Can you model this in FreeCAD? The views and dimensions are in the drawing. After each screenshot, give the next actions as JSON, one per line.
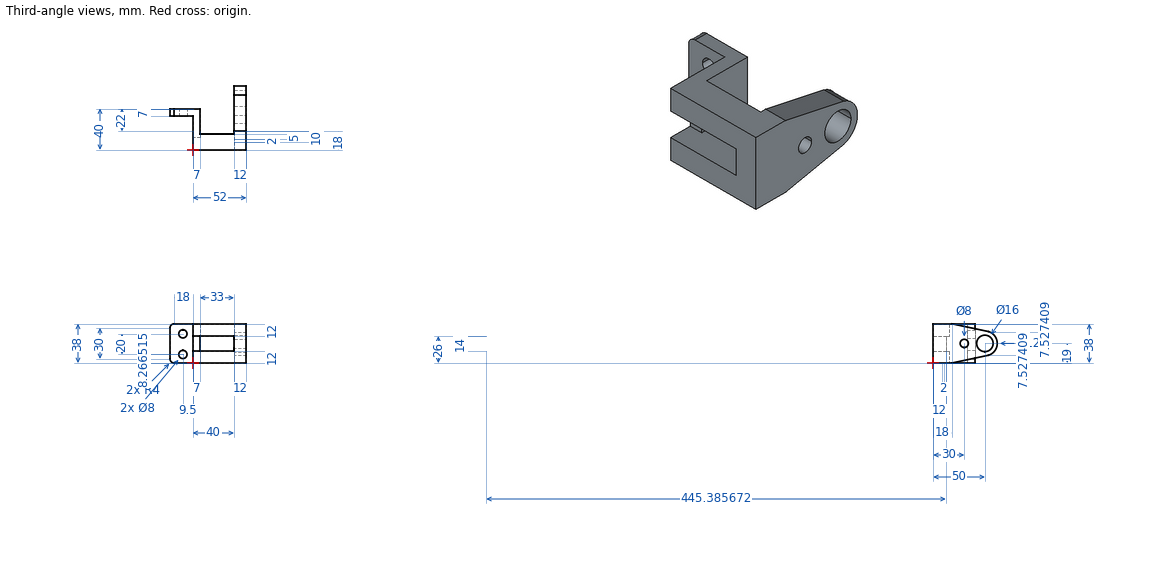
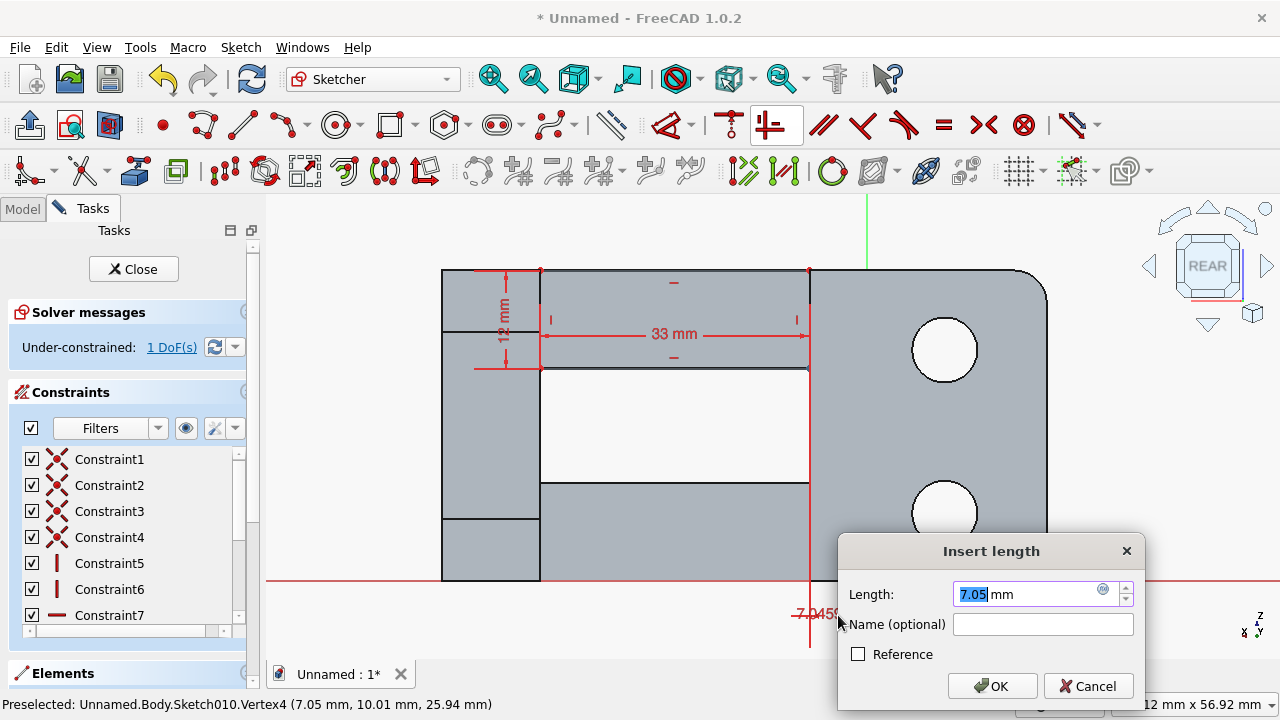
{"action": "type", "text": "7"}
{"action": "key", "text": "Return"}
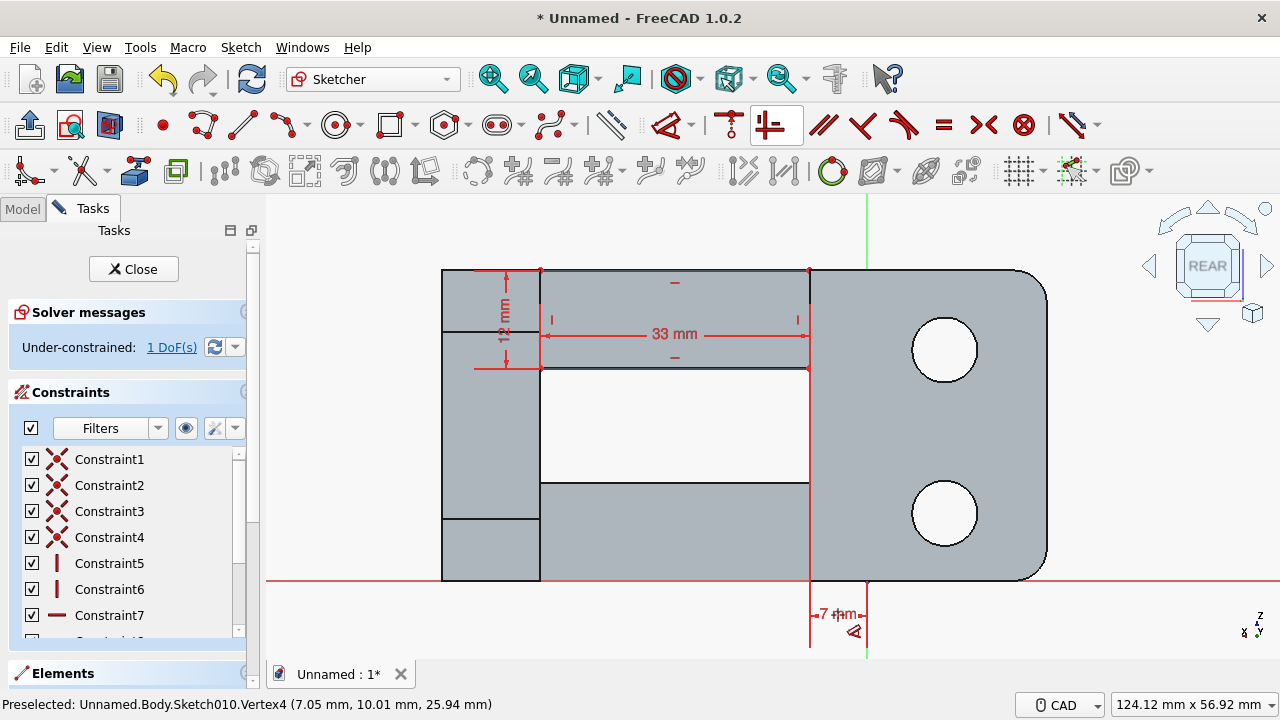
{"action": "left_click", "coordinate": [540, 271]}
{"action": "left_click", "coordinate": [506, 426]}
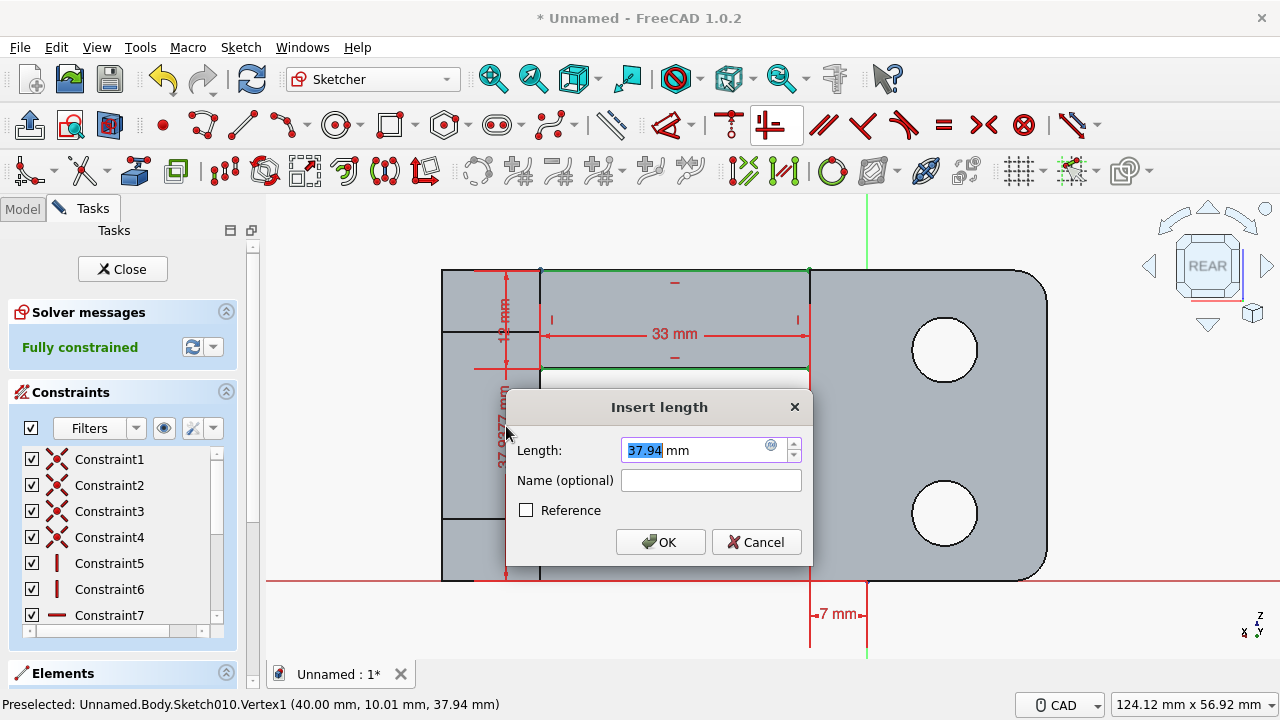
{"action": "type", "text": "38"}
{"action": "key", "text": "Return"}
{"action": "key", "text": "Escape"}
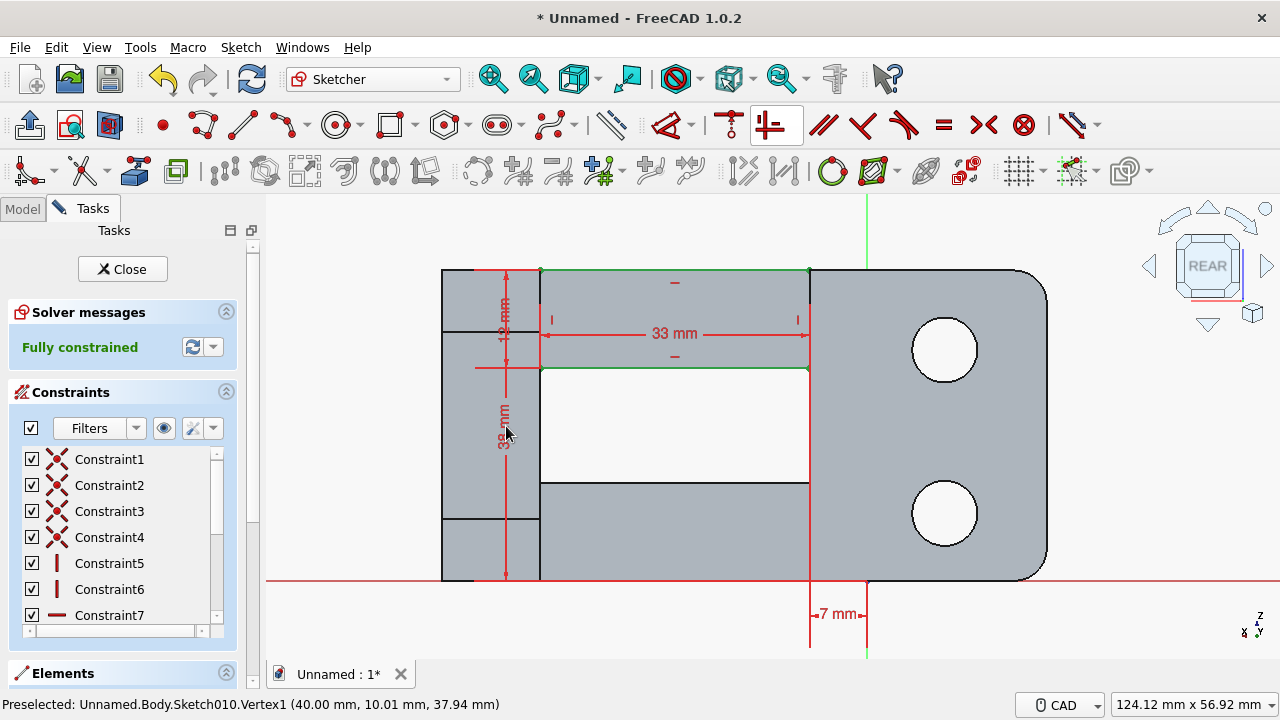
{"action": "left_click", "coordinate": [123, 269]}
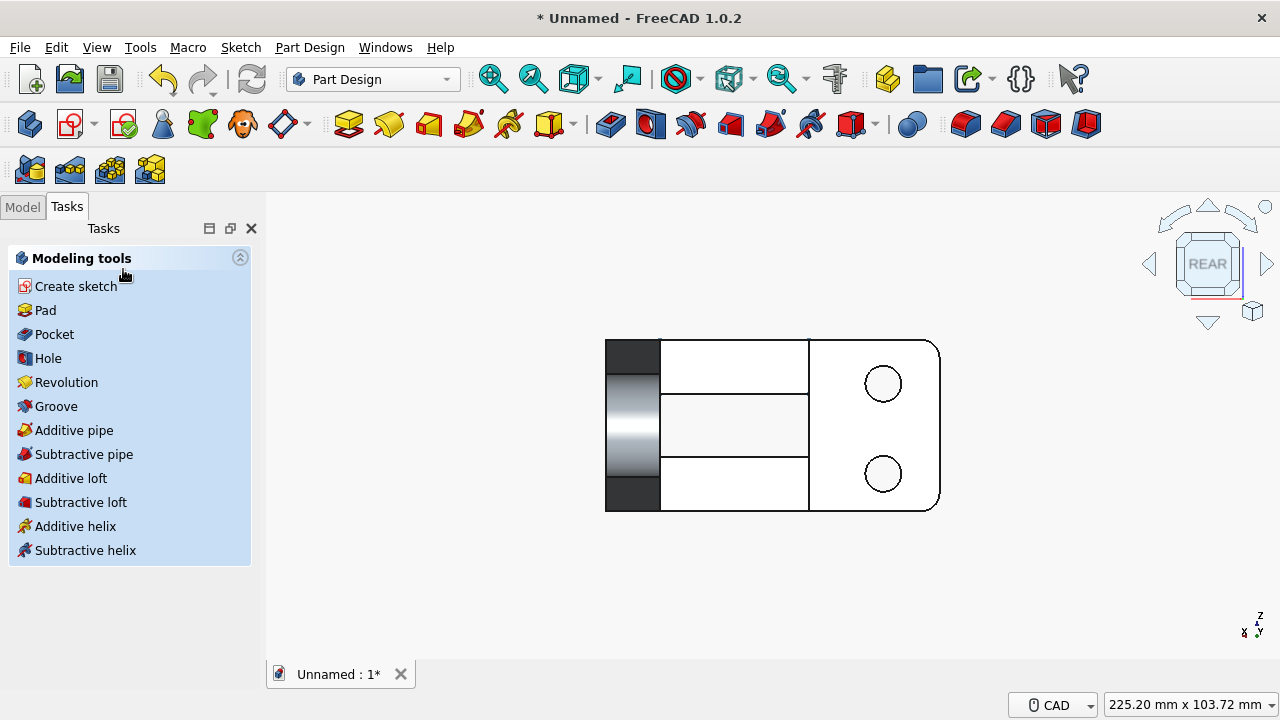
{"action": "left_click", "coordinate": [350, 124]}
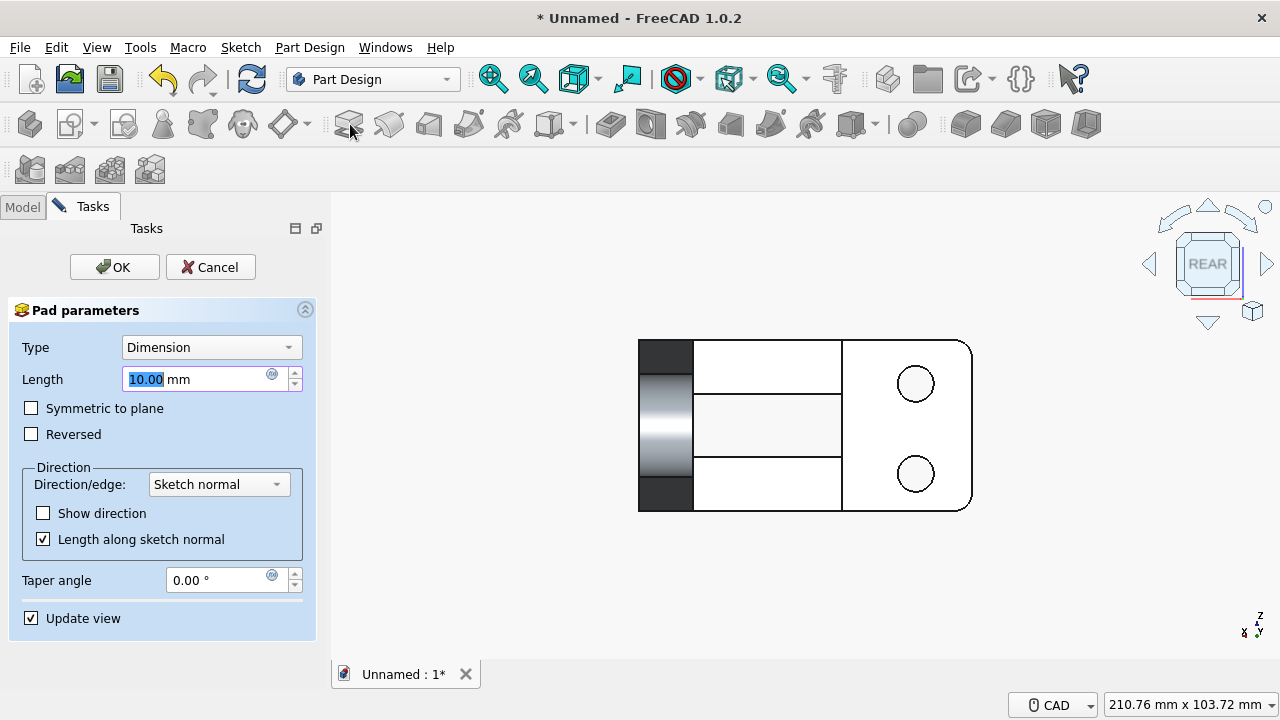
{"action": "type", "text": "5"}
{"action": "key", "text": "Tab"}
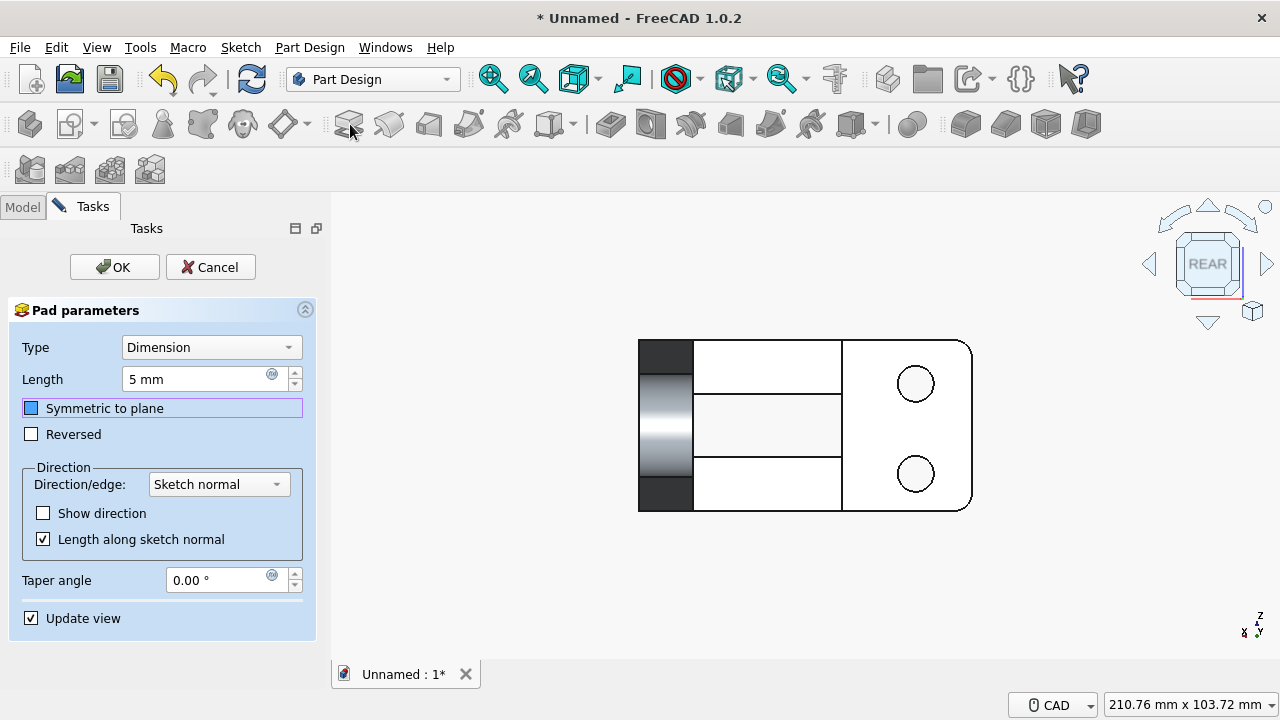
{"action": "left_click", "coordinate": [115, 267]}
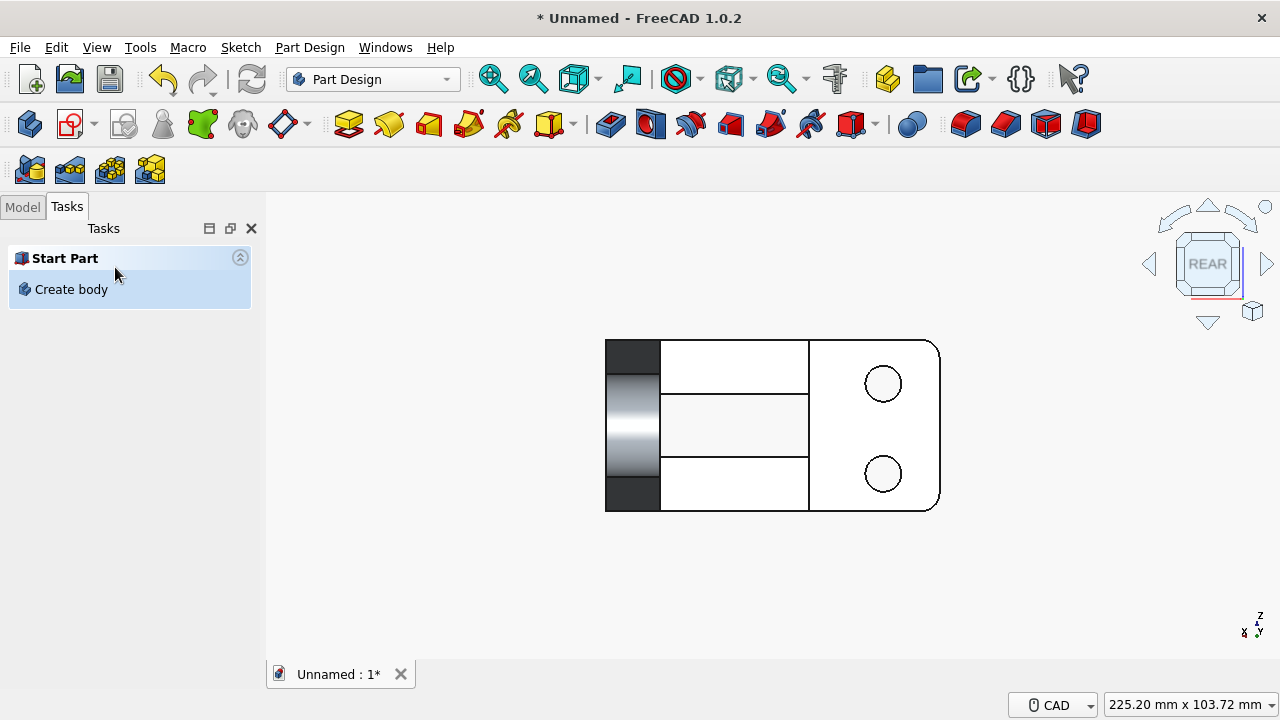
{"action": "left_click", "coordinate": [494, 80]}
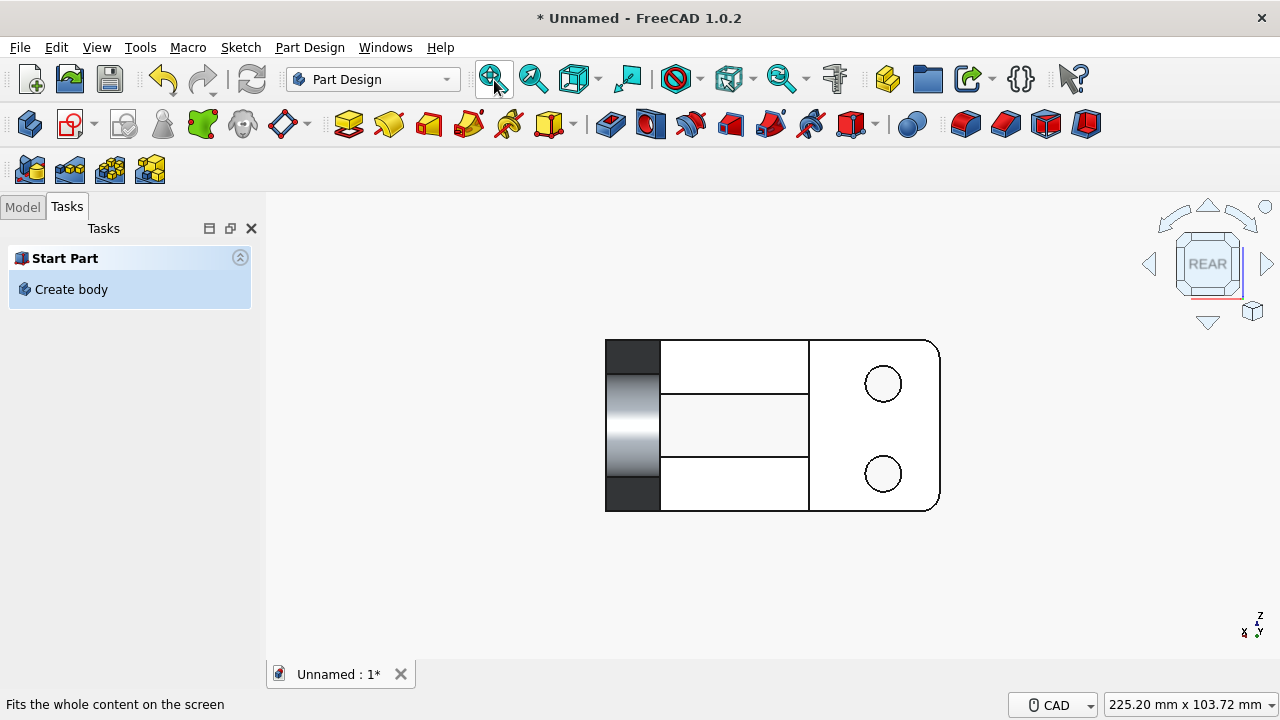
{"action": "left_click", "coordinate": [692, 483]}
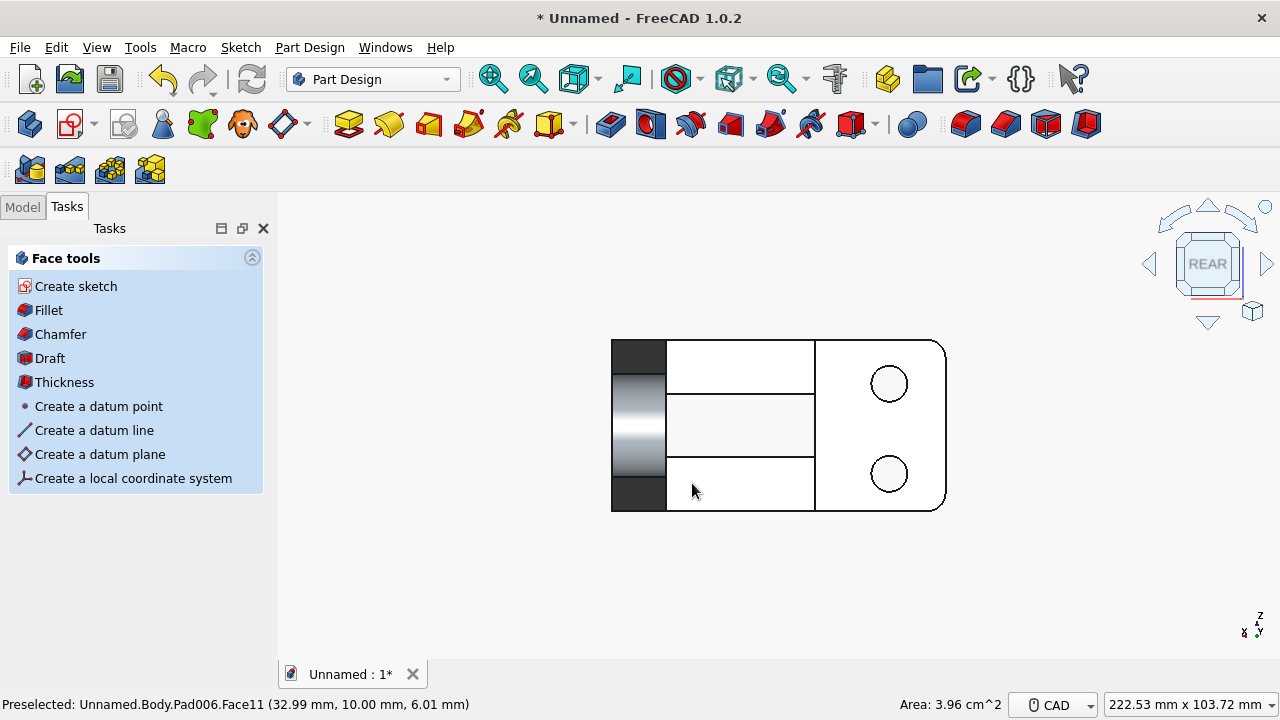
{"action": "left_click", "coordinate": [70, 124]}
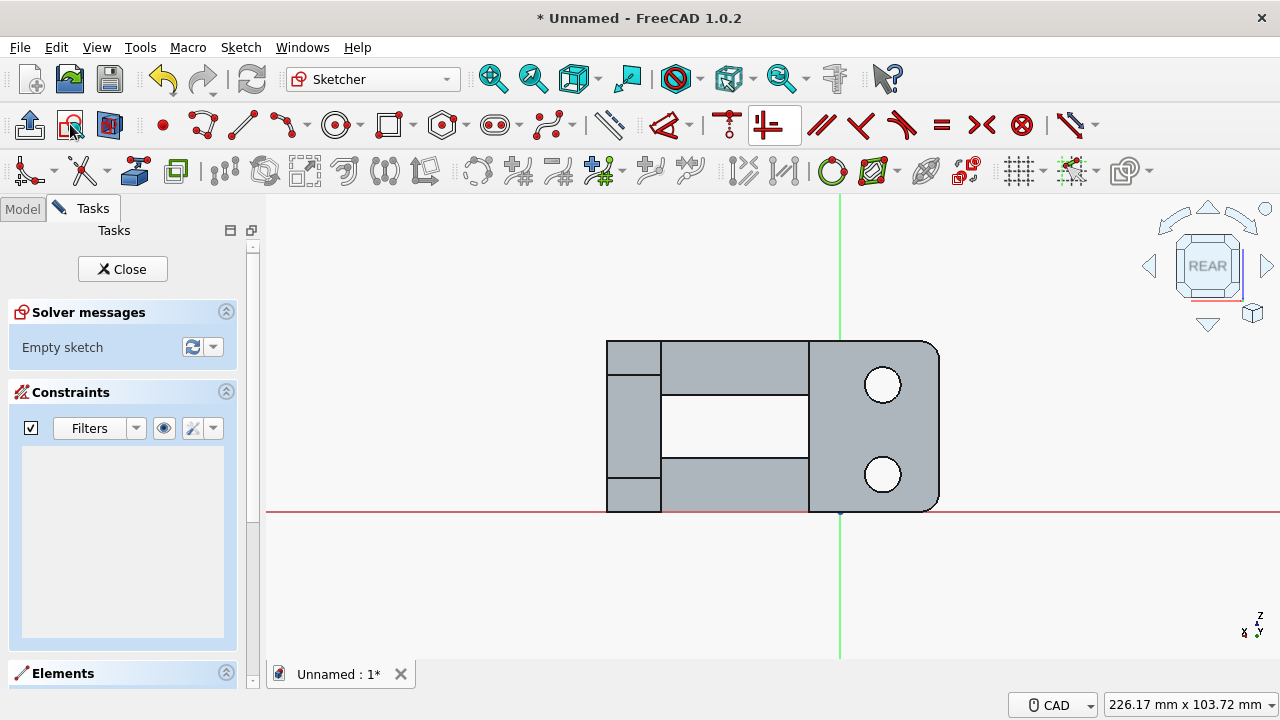
{"action": "left_click", "coordinate": [110, 126]}